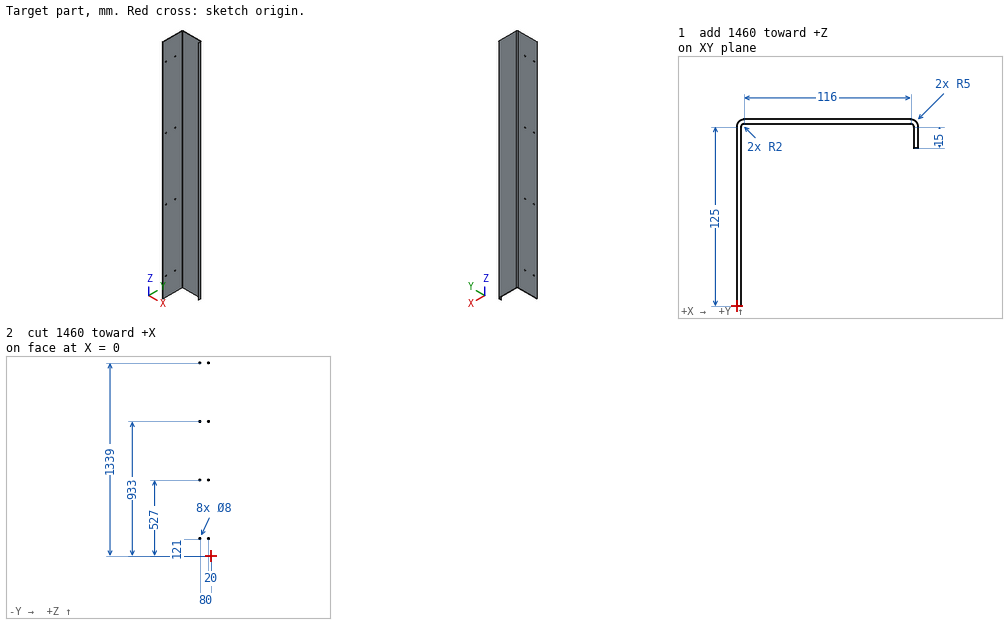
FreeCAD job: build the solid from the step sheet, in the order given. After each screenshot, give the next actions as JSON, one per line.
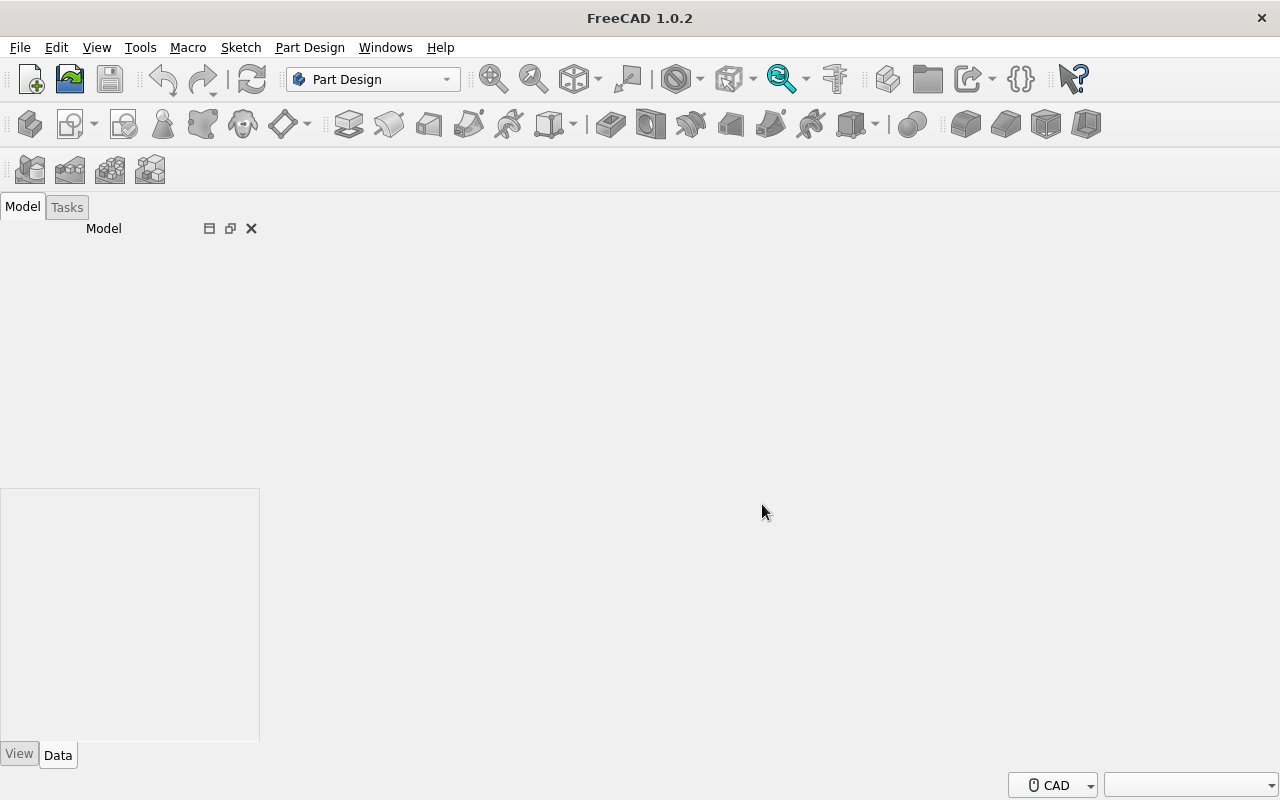
{"action": "left_click", "coordinate": [30, 80]}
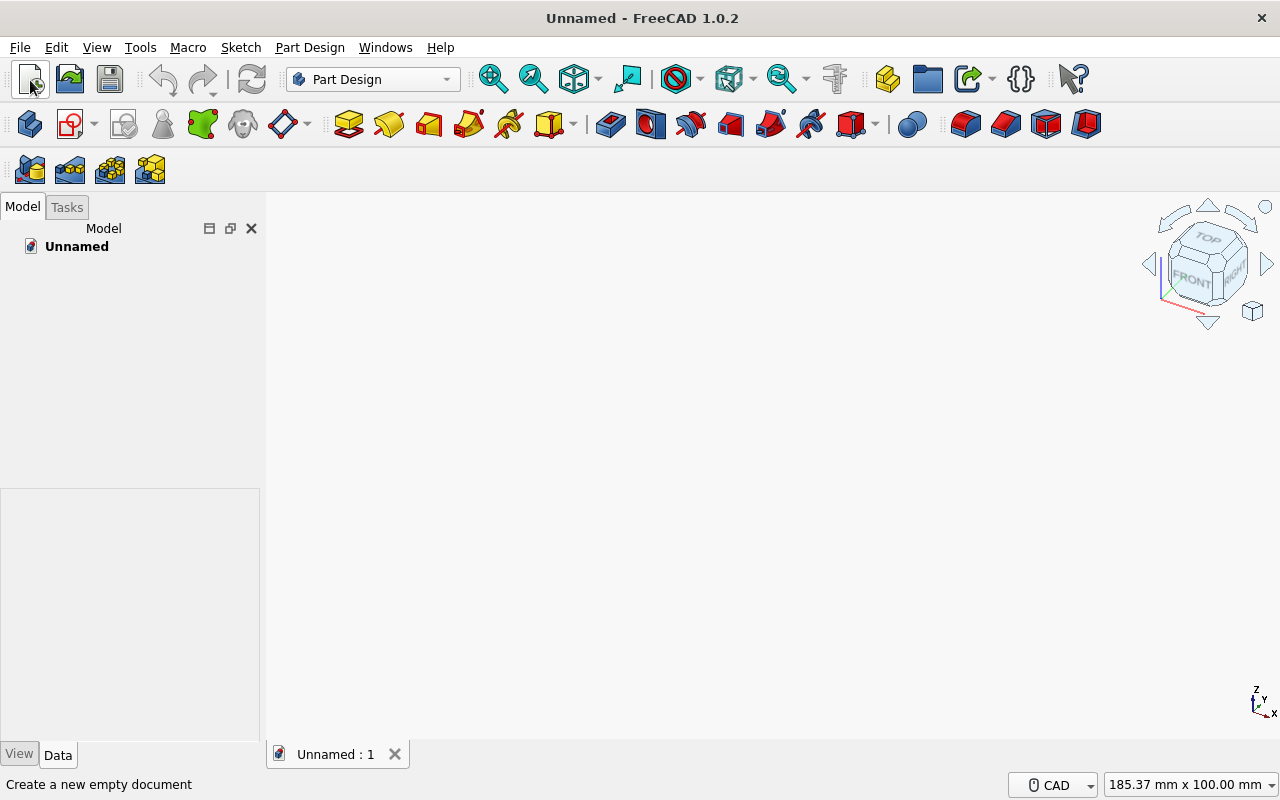
{"action": "left_click", "coordinate": [70, 124]}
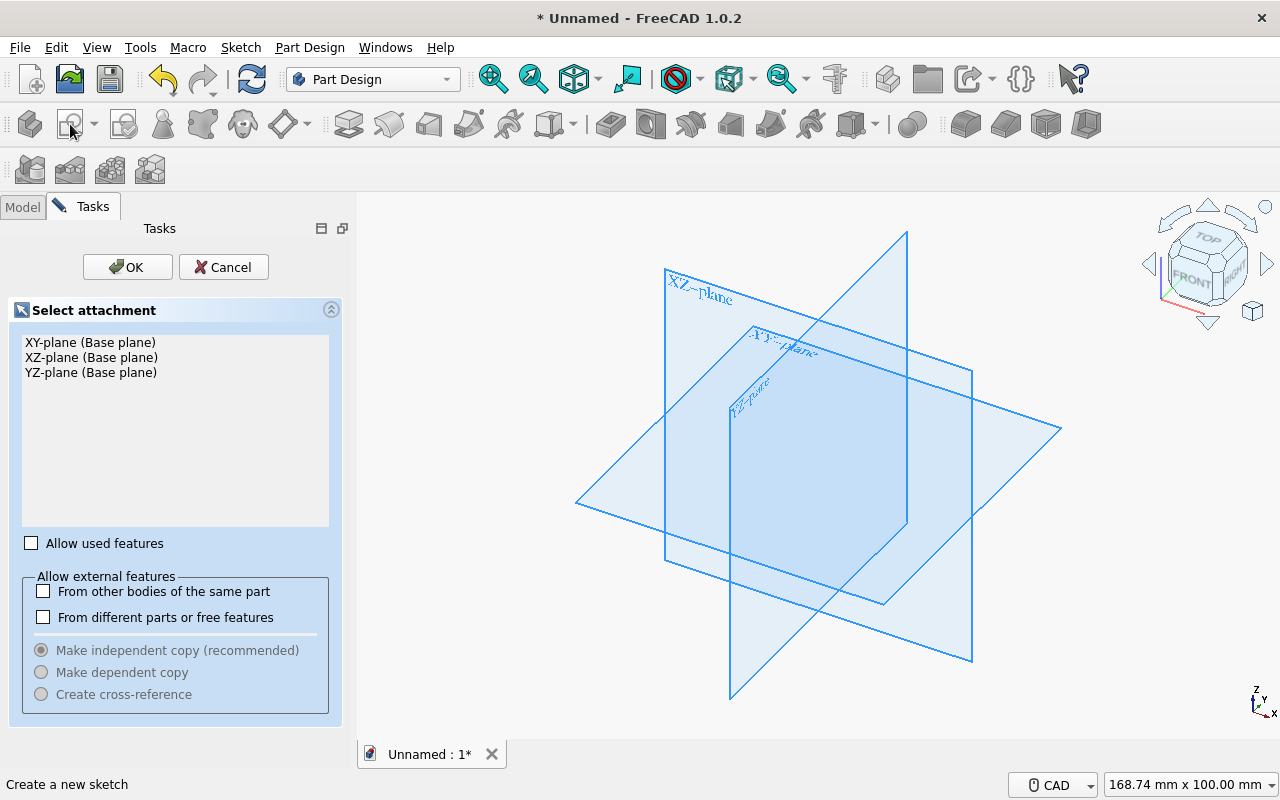
{"action": "left_click", "coordinate": [82, 342]}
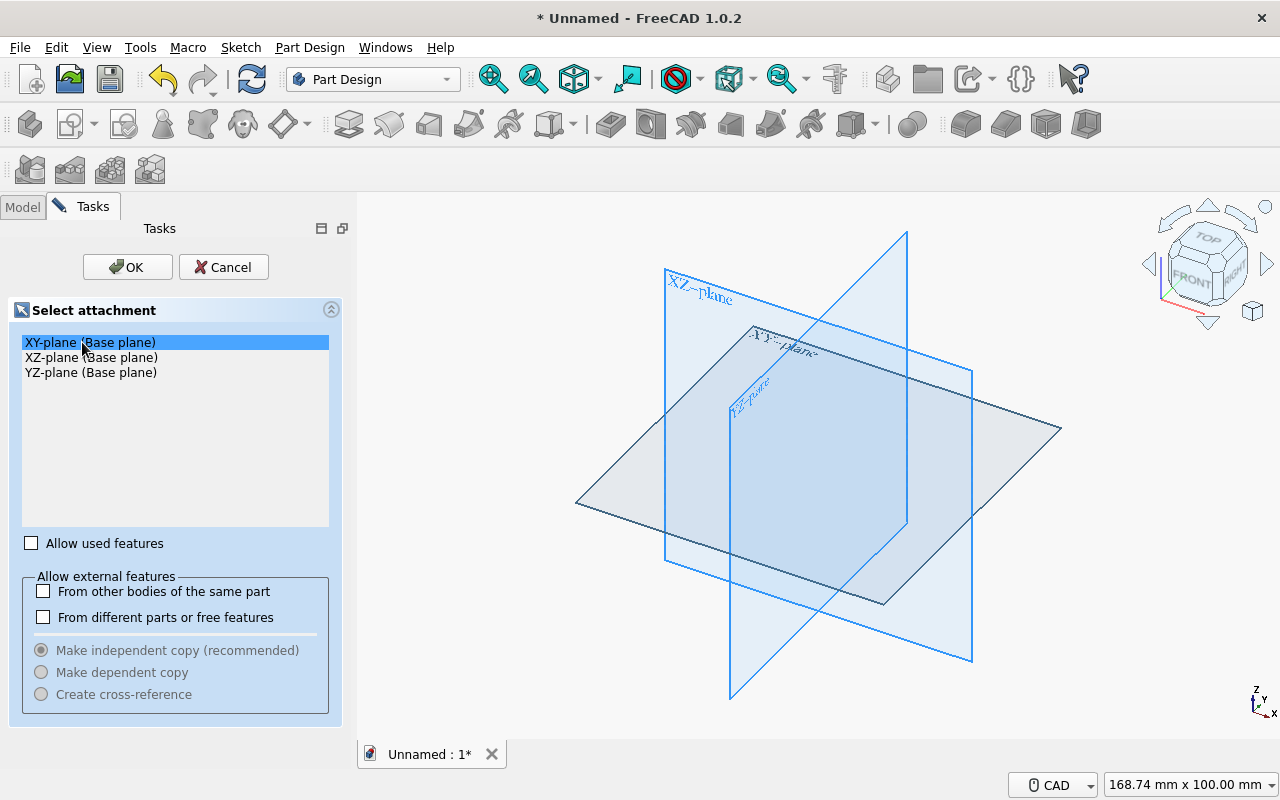
{"action": "left_click", "coordinate": [128, 267]}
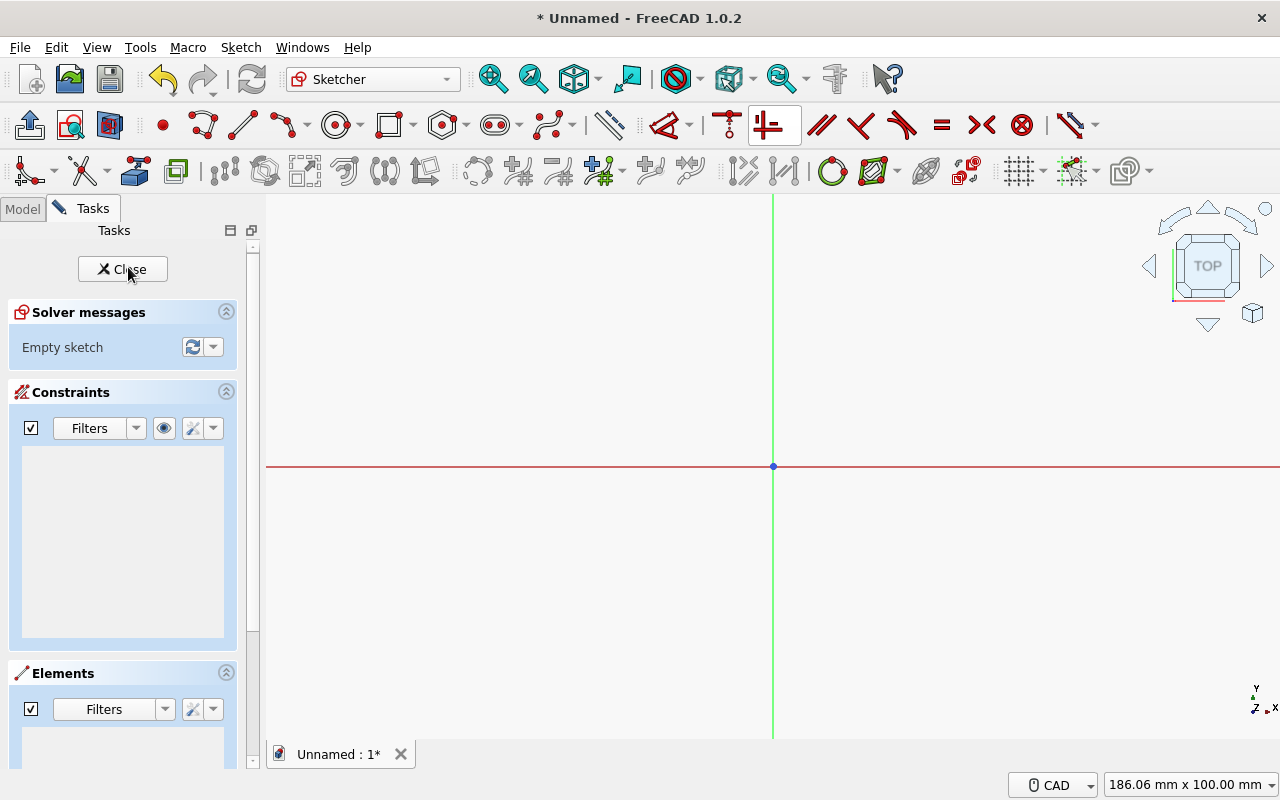
{"action": "scroll", "coordinate": [368, 711], "scroll_direction": "down", "scroll_amount": 4}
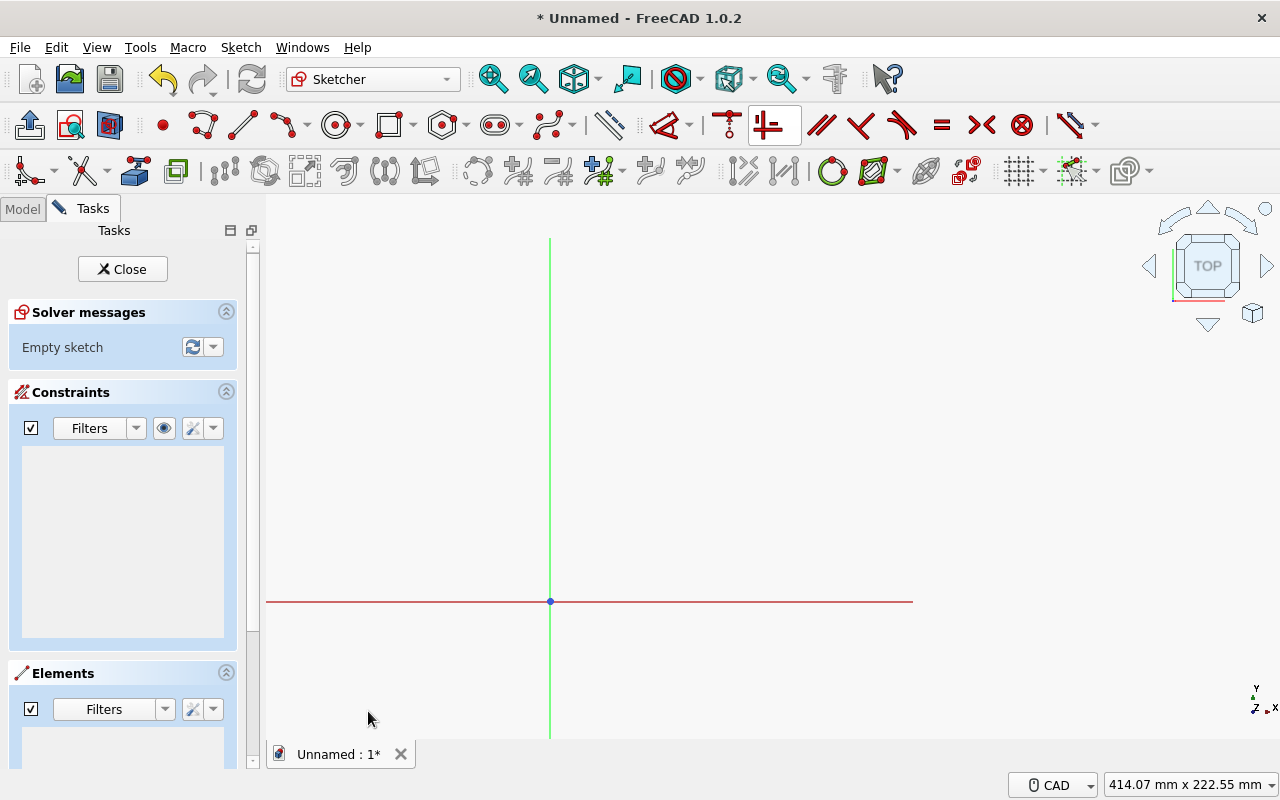
{"action": "left_click", "coordinate": [204, 126]}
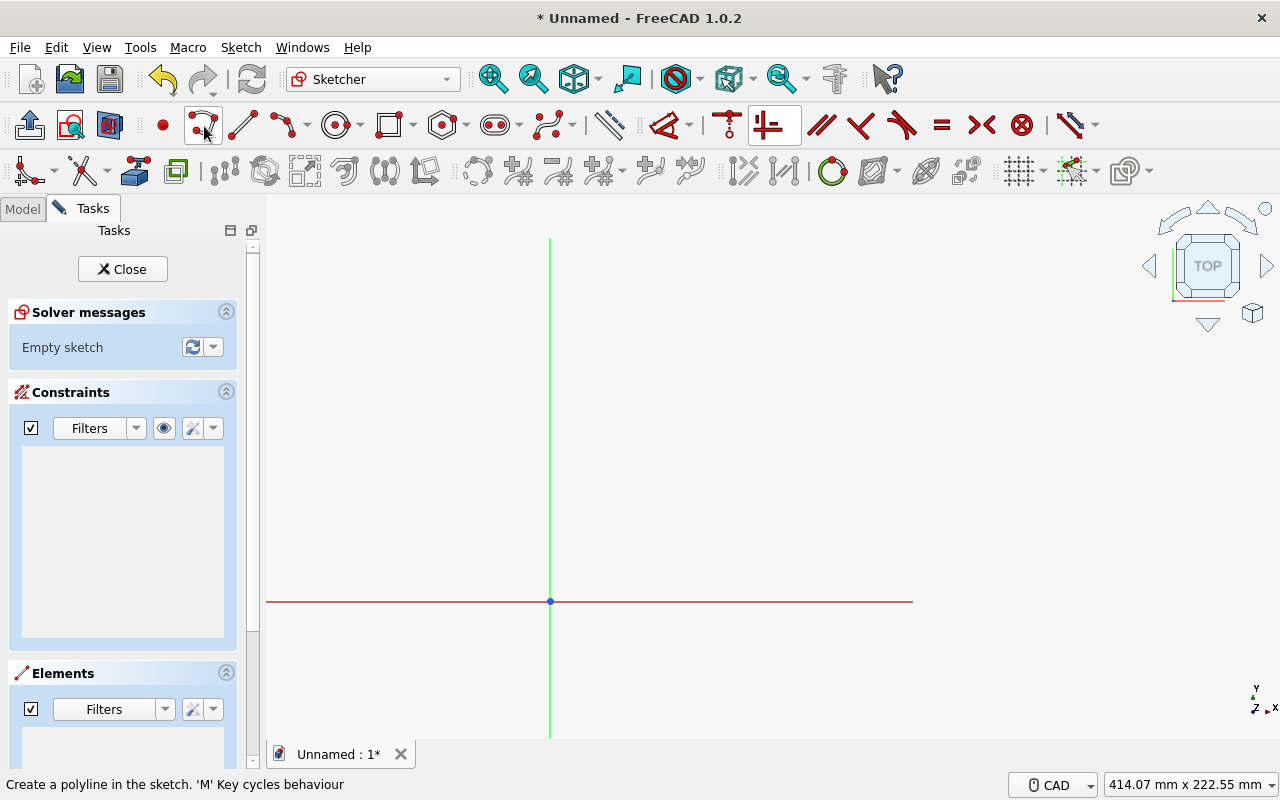
{"action": "left_click", "coordinate": [550, 296]}
{"action": "left_click", "coordinate": [550, 602]}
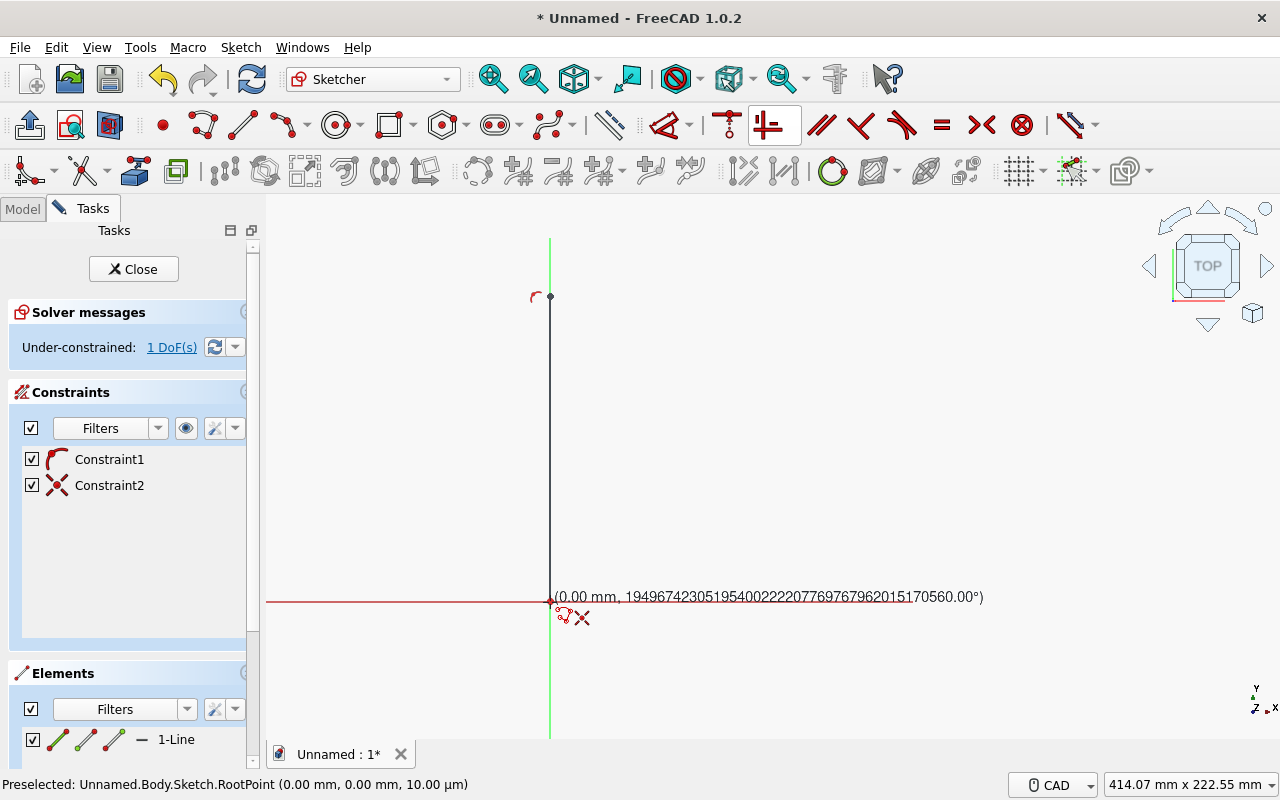
{"action": "scroll", "coordinate": [557, 602], "scroll_direction": "up", "scroll_amount": 4}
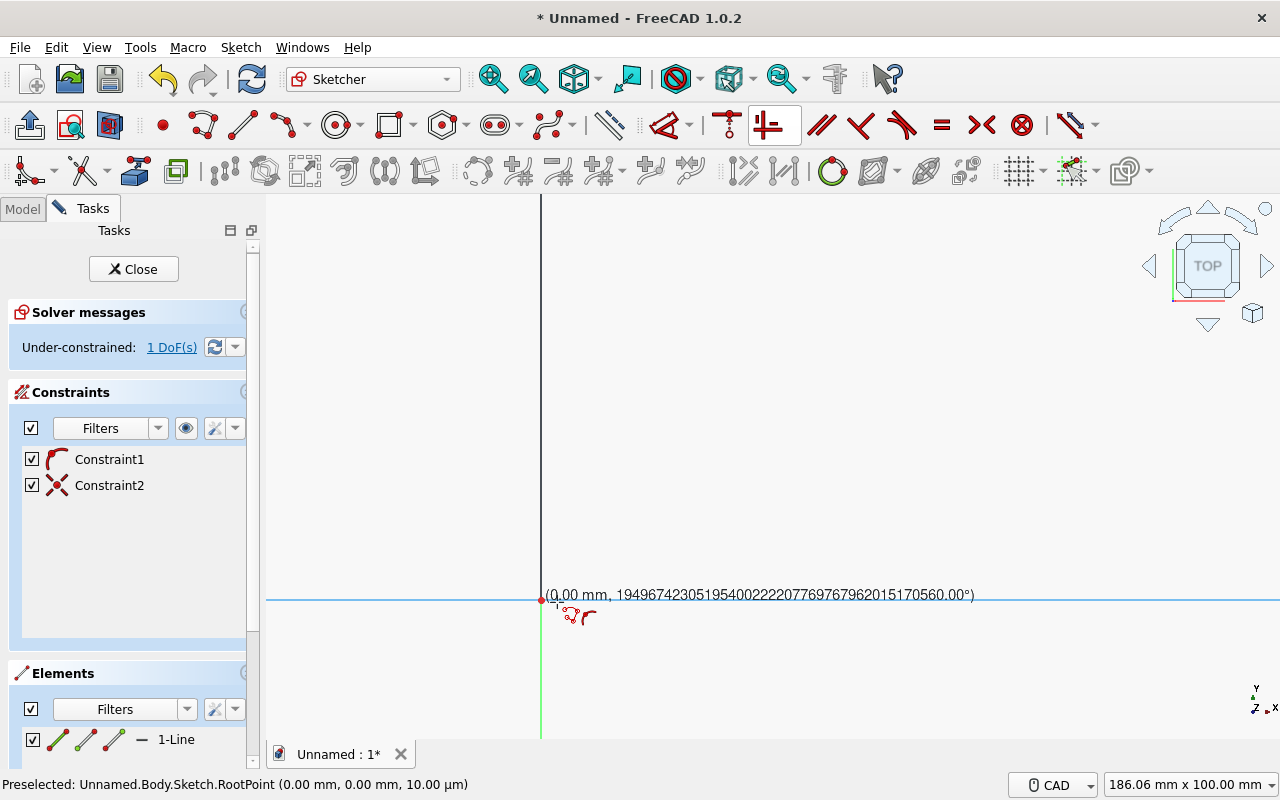
{"action": "left_click", "coordinate": [557, 591]}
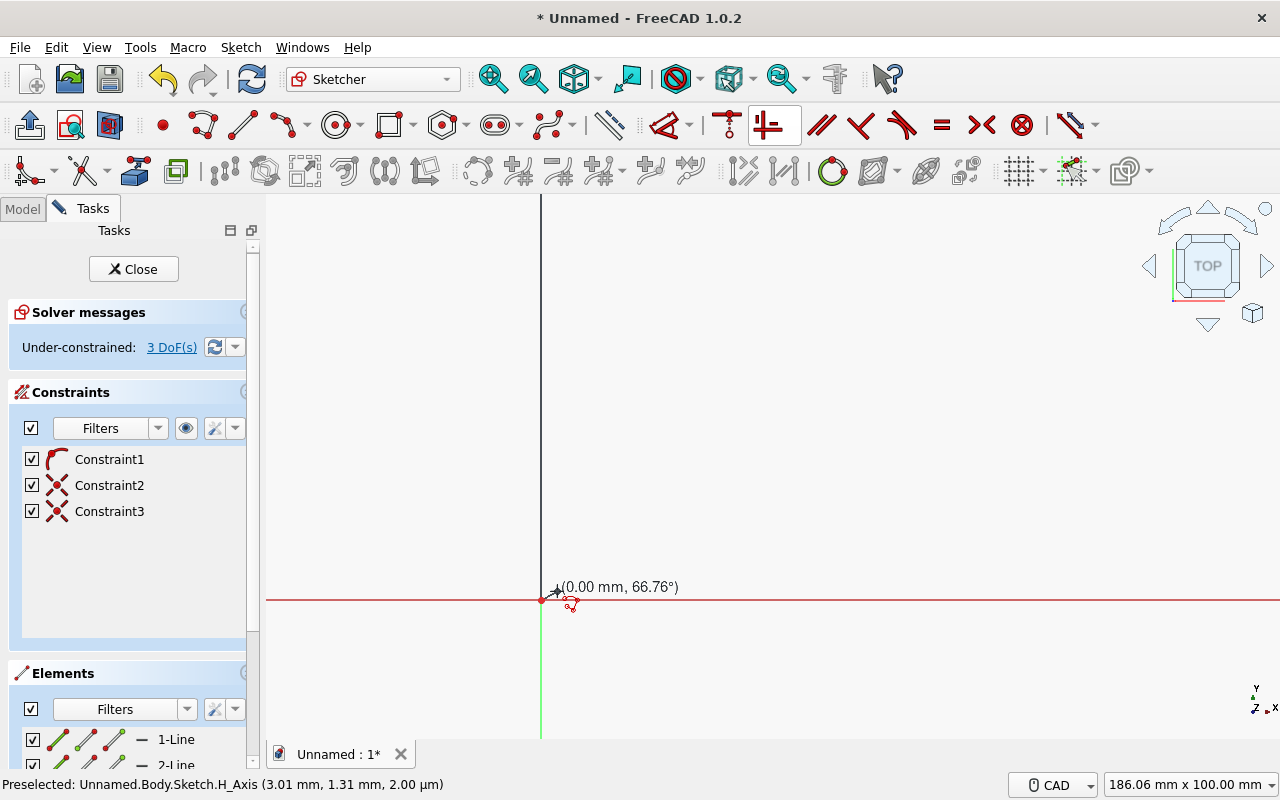
{"action": "scroll", "coordinate": [558, 646], "scroll_direction": "down", "scroll_amount": 4}